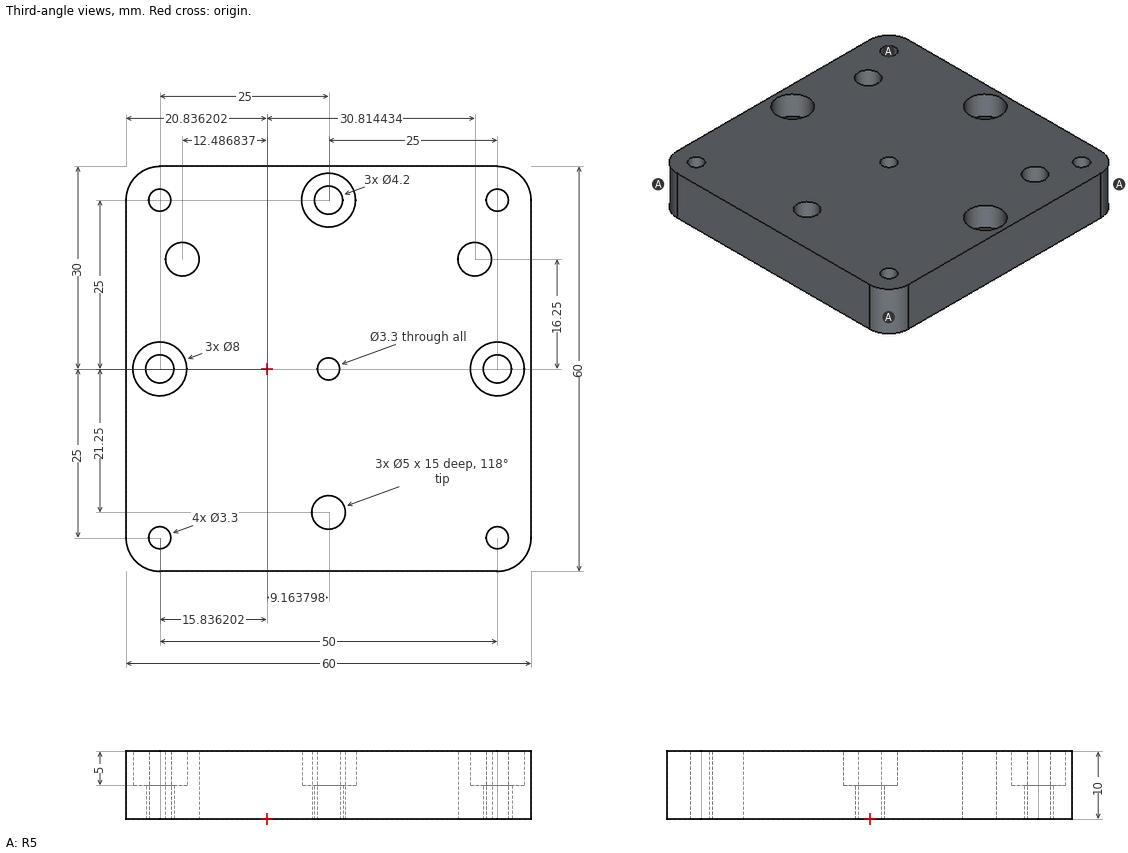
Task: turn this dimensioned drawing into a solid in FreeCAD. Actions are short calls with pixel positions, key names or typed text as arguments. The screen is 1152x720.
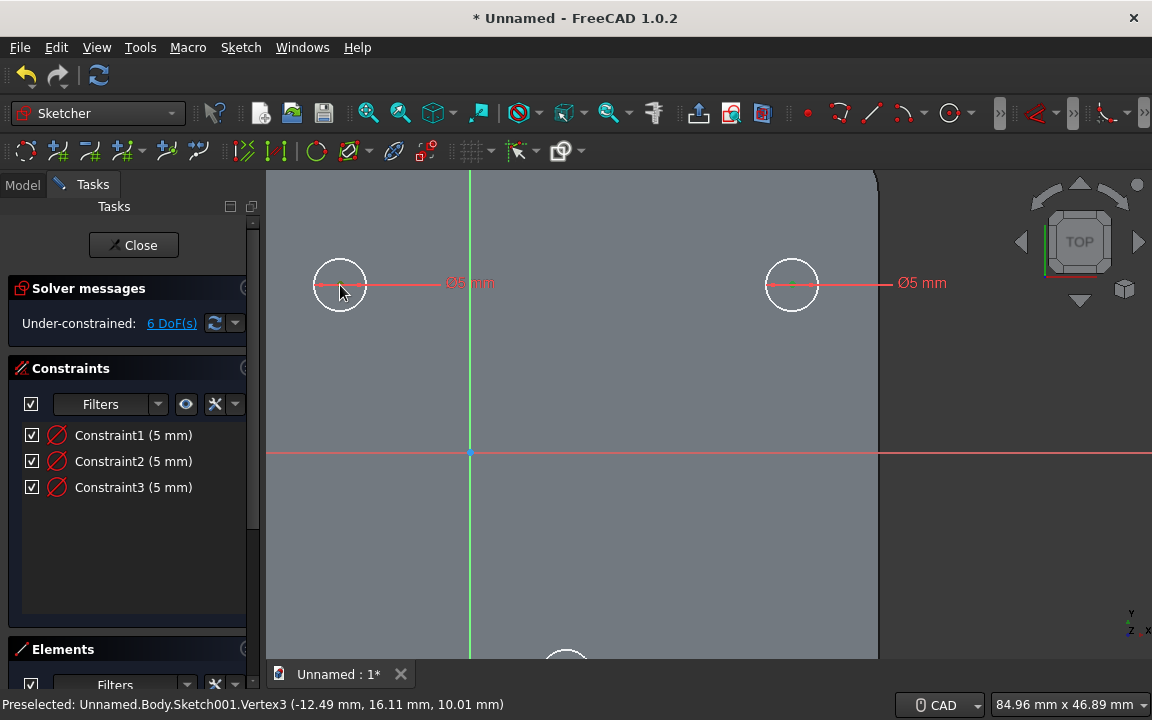
key(h)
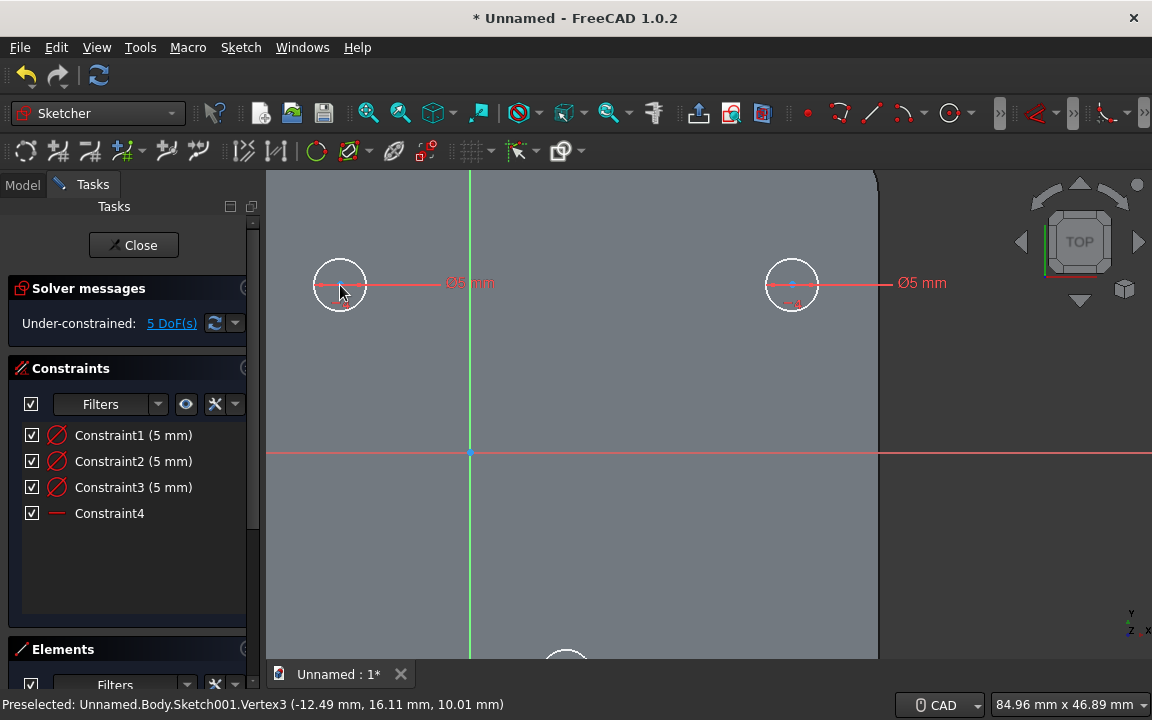
click(1036, 114)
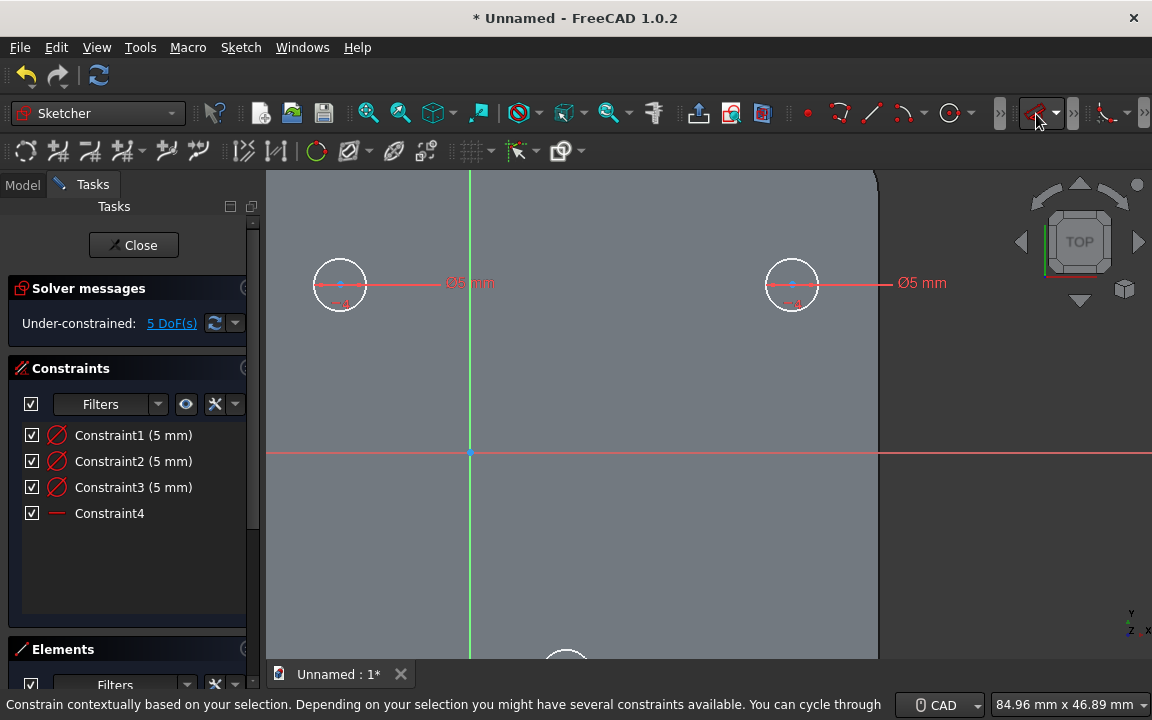
scroll(792, 283, down, 2)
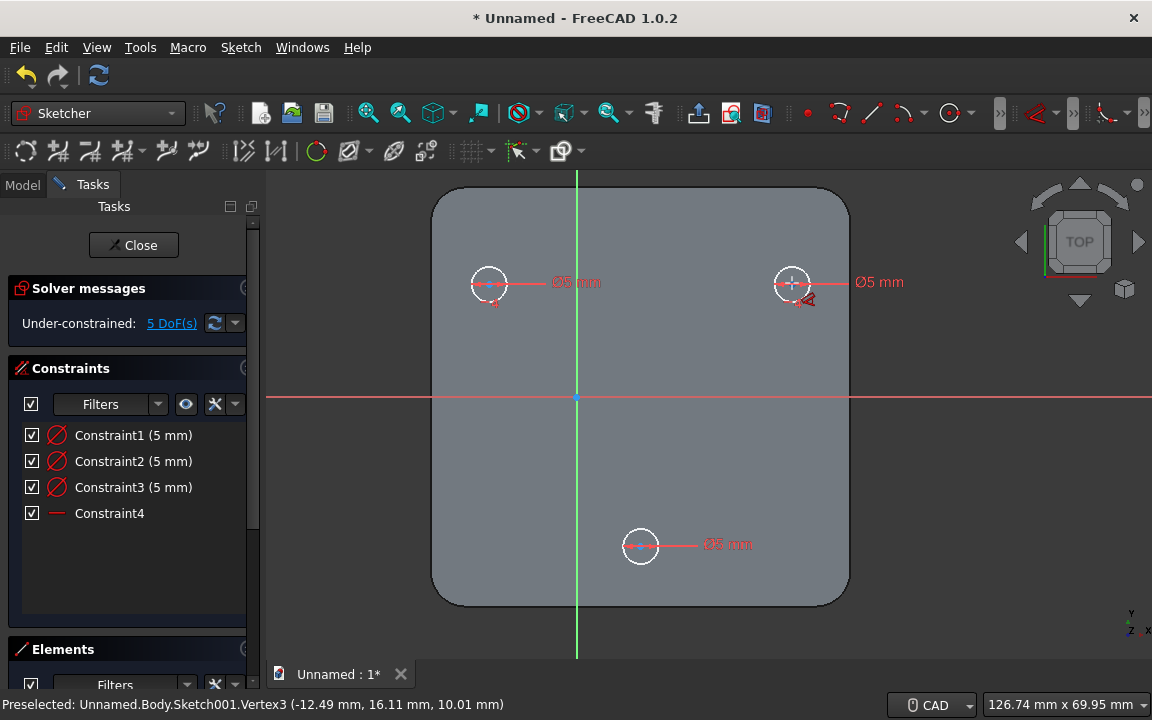
click(641, 546)
click(543, 472)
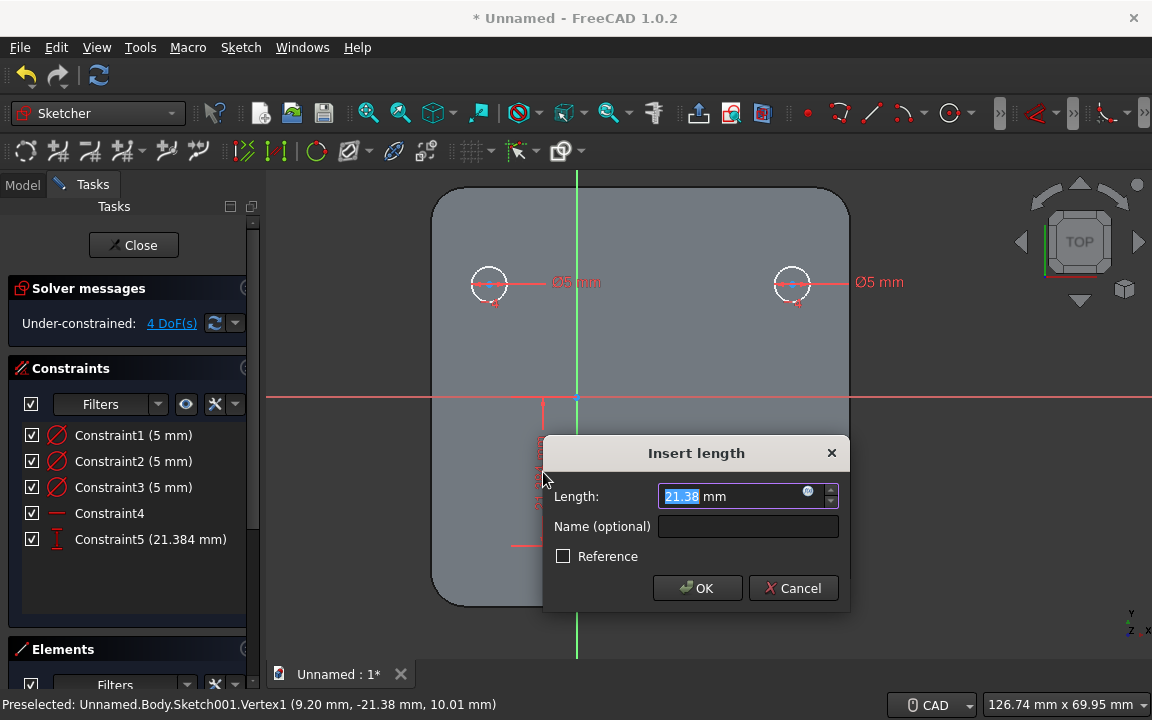
text(21.25)
key(Return)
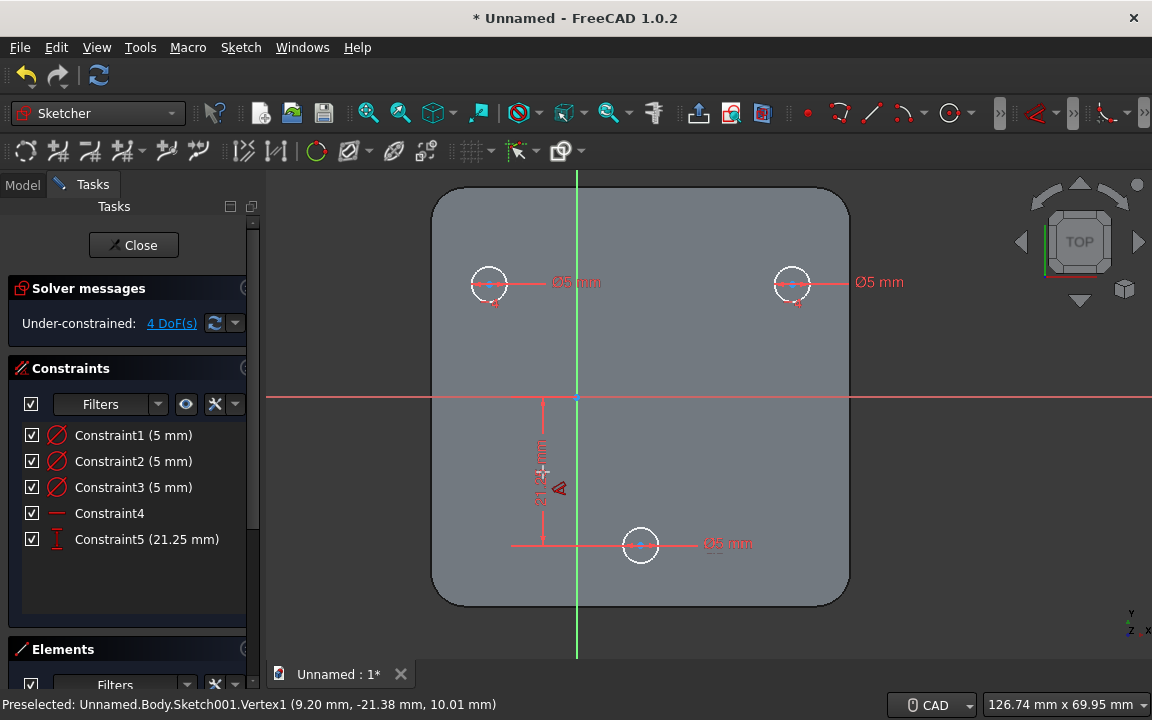
click(792, 284)
click(826, 341)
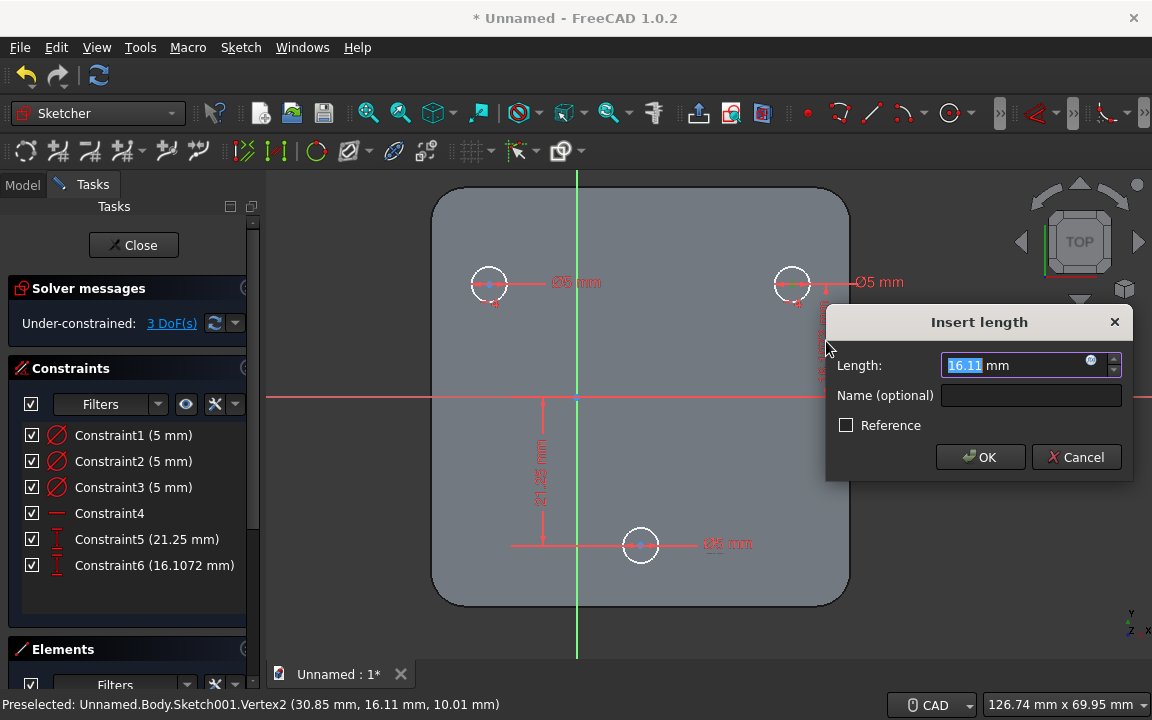
text(16.25)
key(Return)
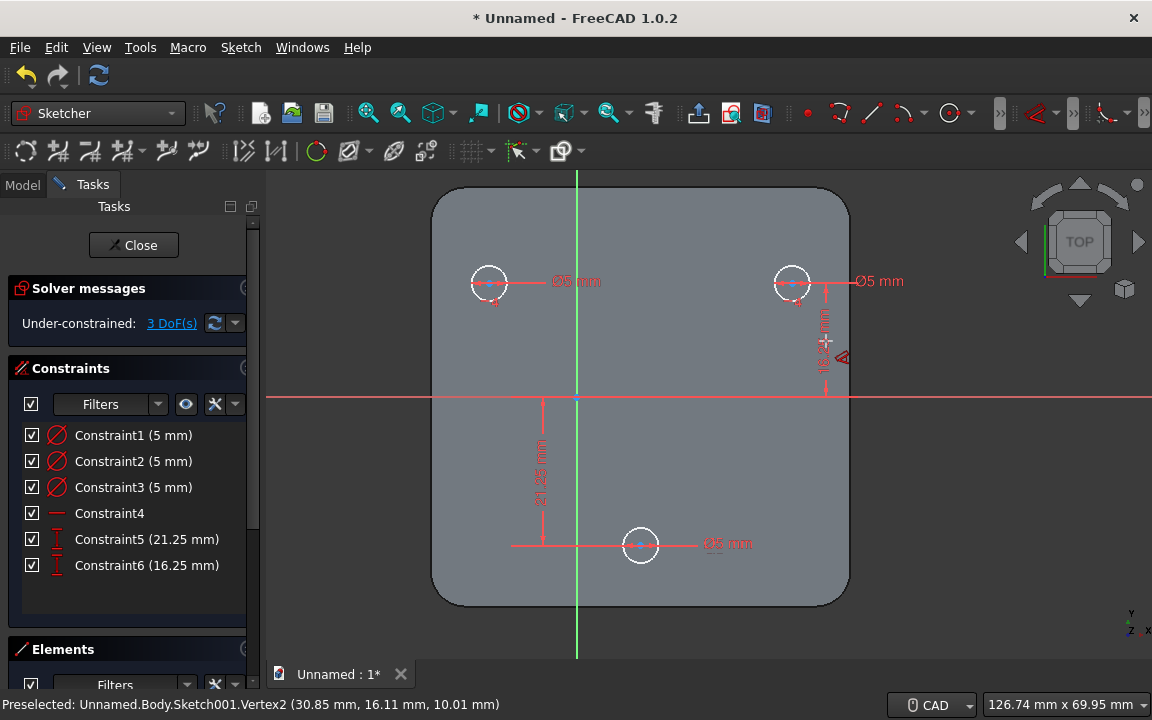
click(641, 546)
click(609, 580)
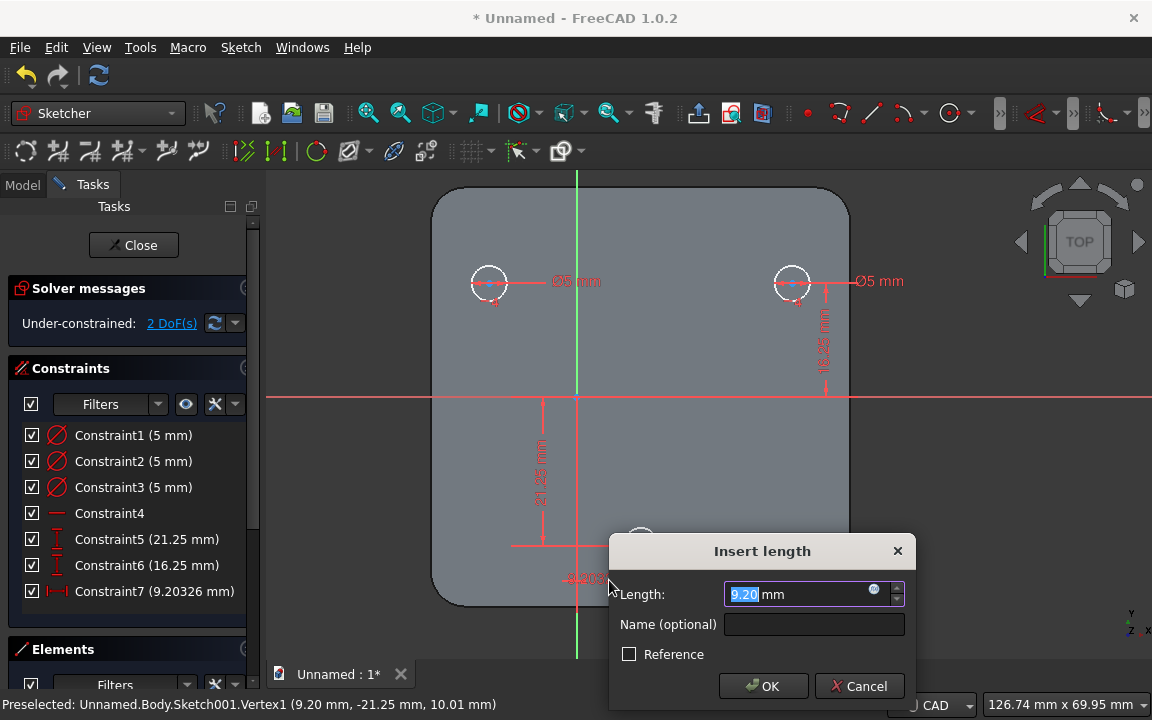
text(9.163798)
key(Return)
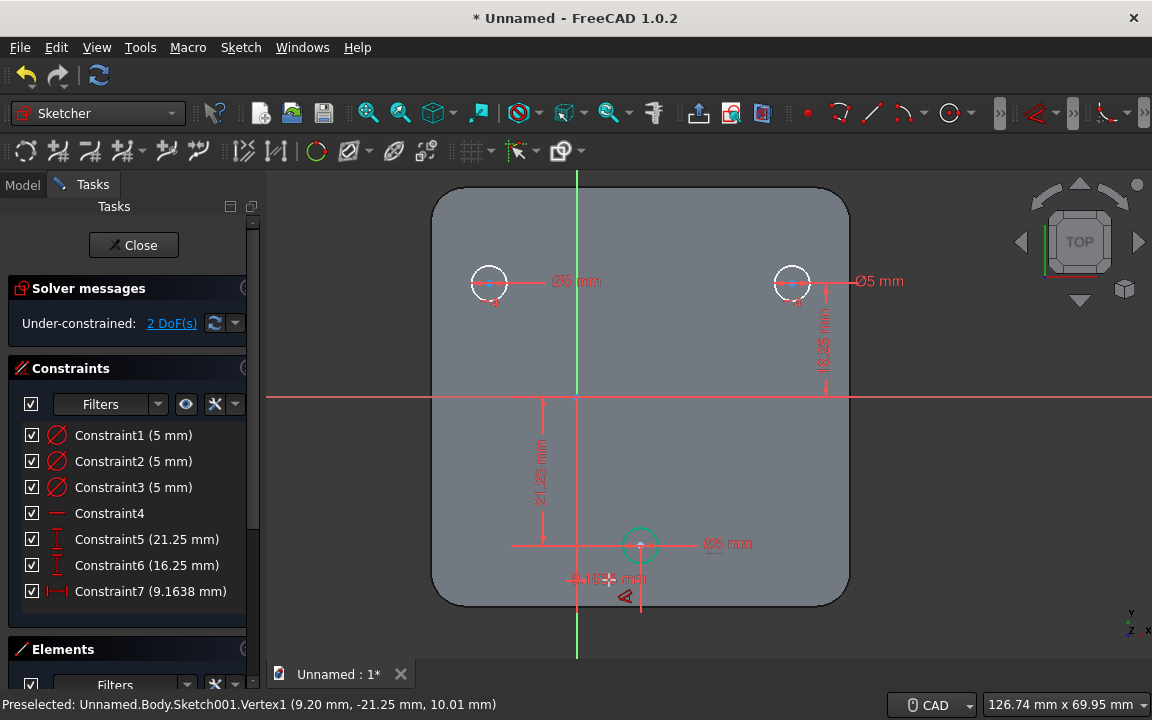
click(792, 283)
click(684, 249)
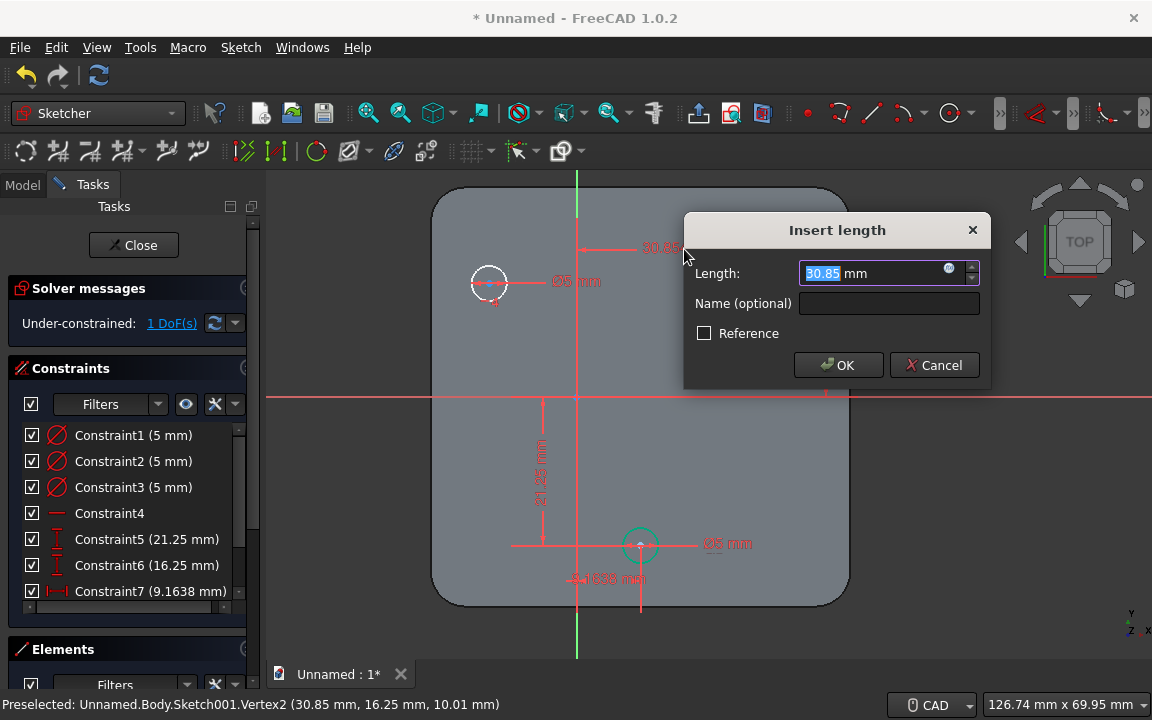
text(30.814434)
key(Return)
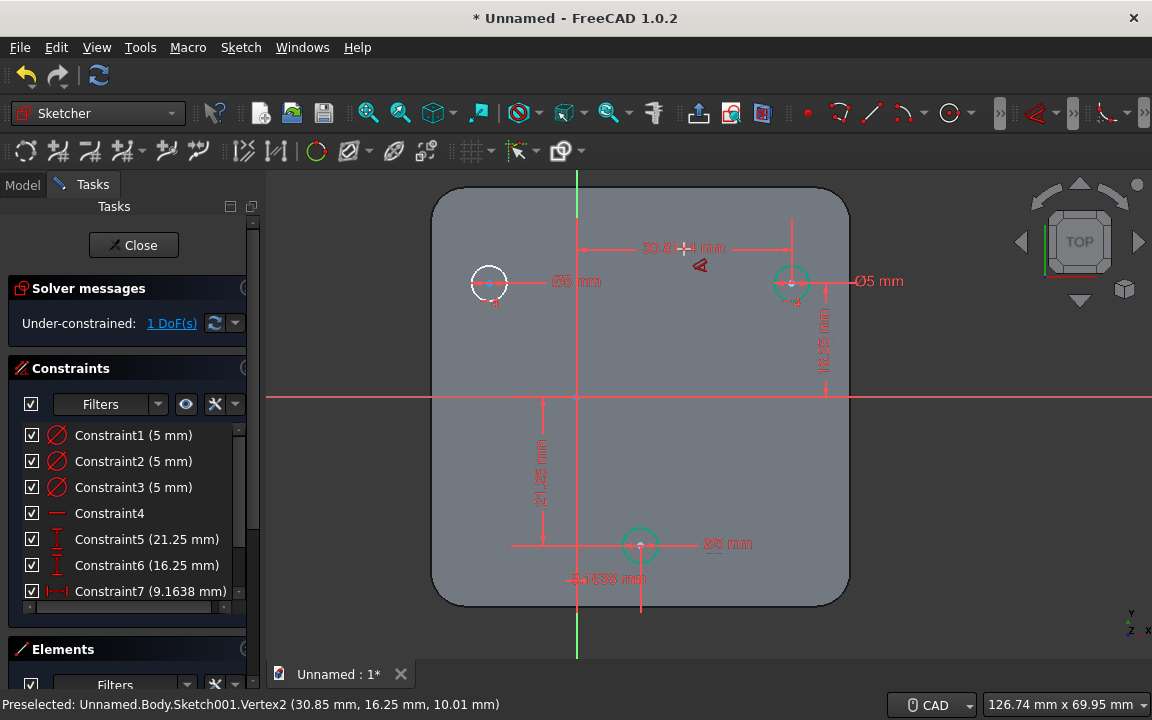
click(489, 283)
click(533, 249)